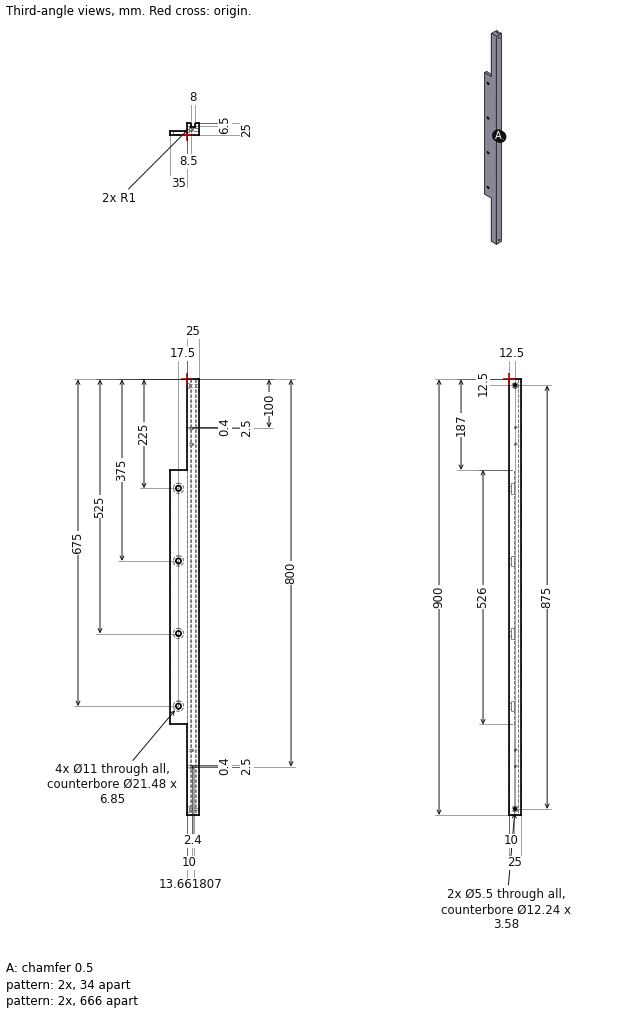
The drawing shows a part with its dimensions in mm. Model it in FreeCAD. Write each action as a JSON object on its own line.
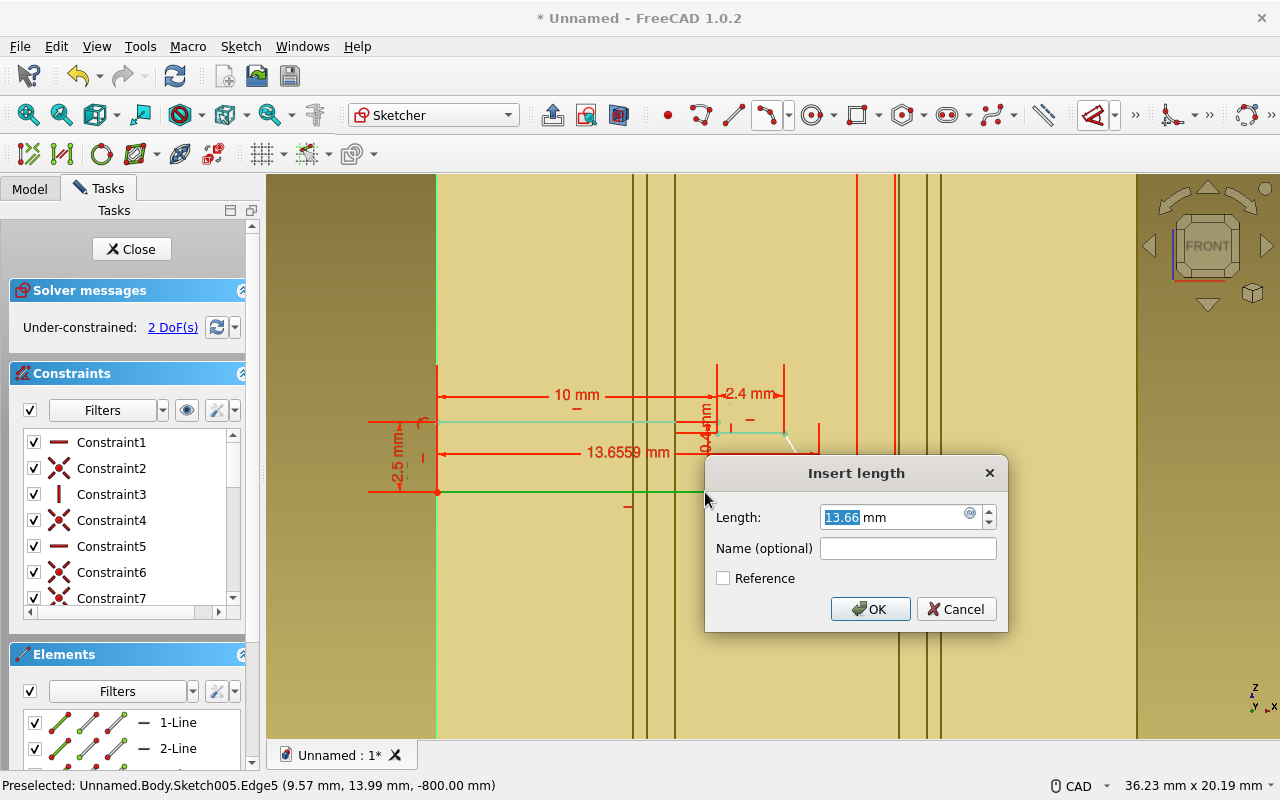
{"action": "type", "text": "13.661807"}
{"action": "key", "text": "Return"}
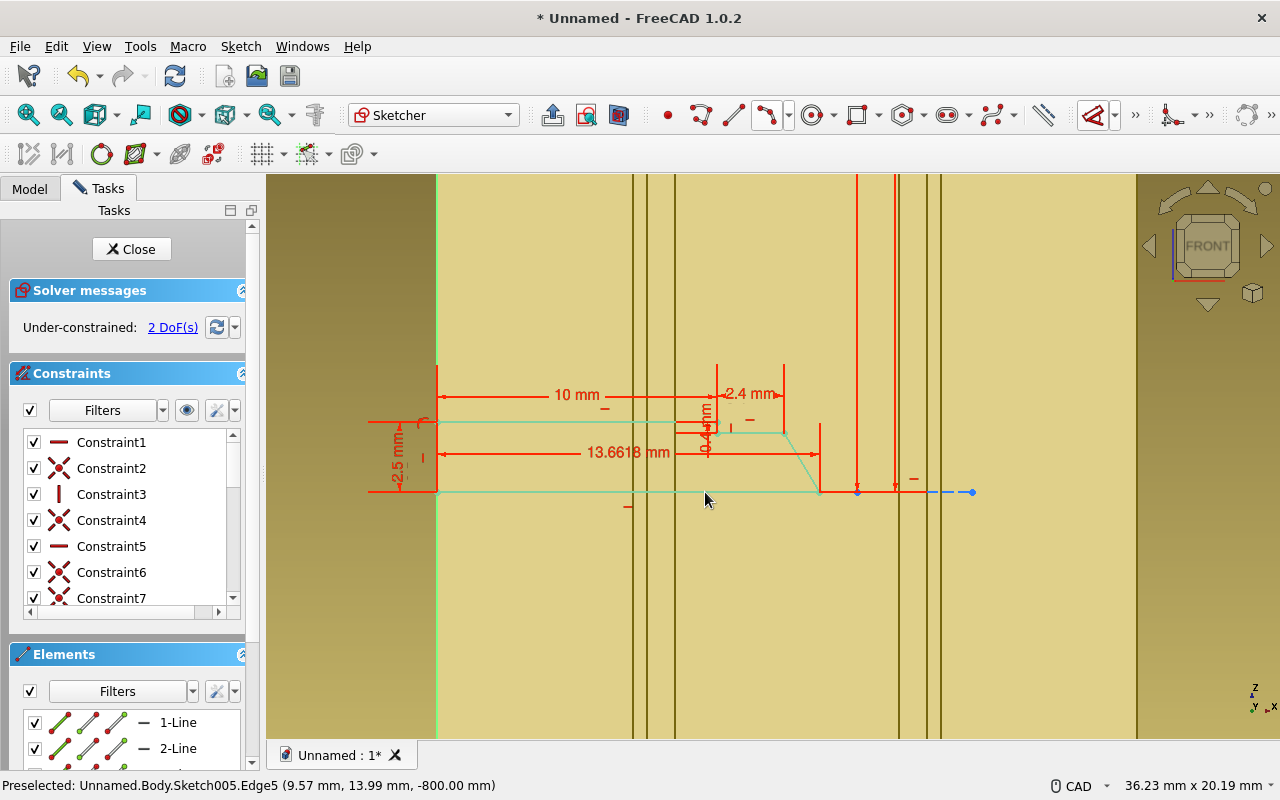
{"action": "left_click", "coordinate": [132, 249]}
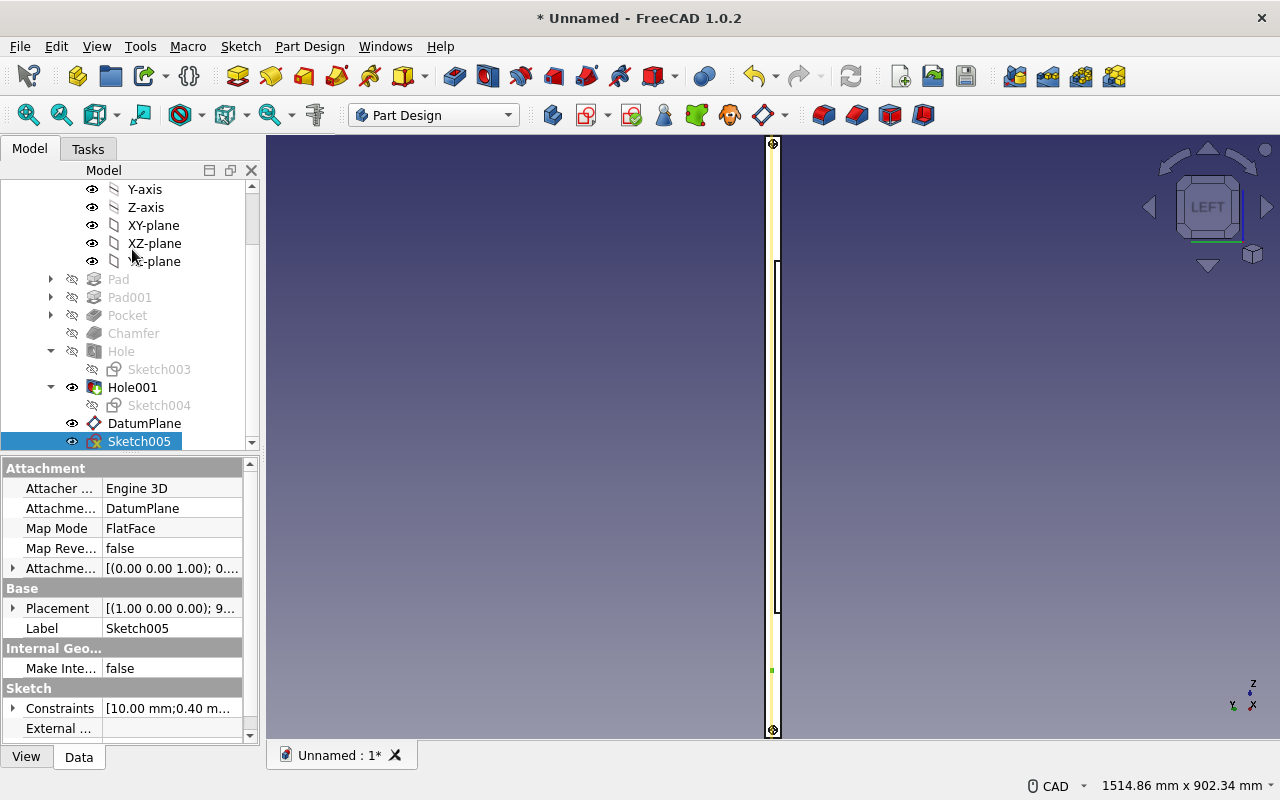
{"action": "left_click", "coordinate": [521, 76]}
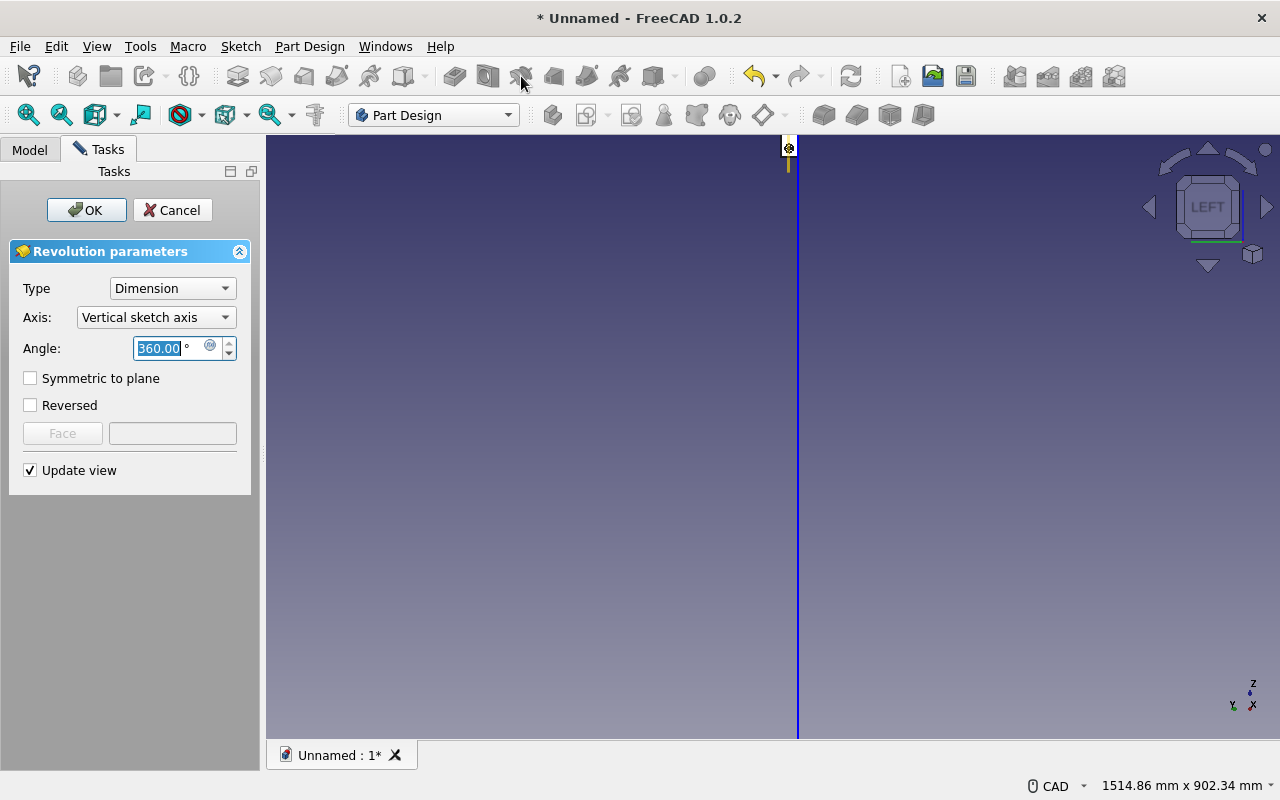
{"action": "left_click", "coordinate": [157, 318]}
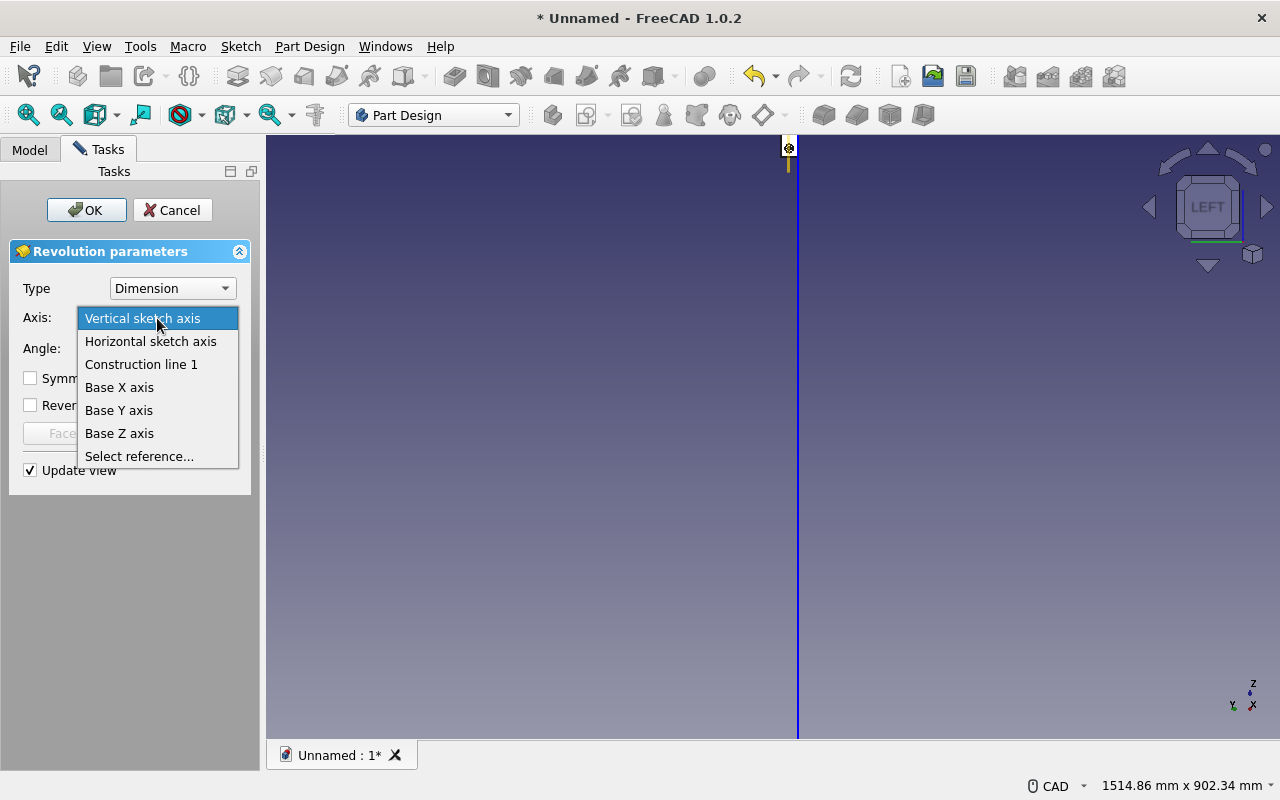
{"action": "left_click", "coordinate": [156, 364]}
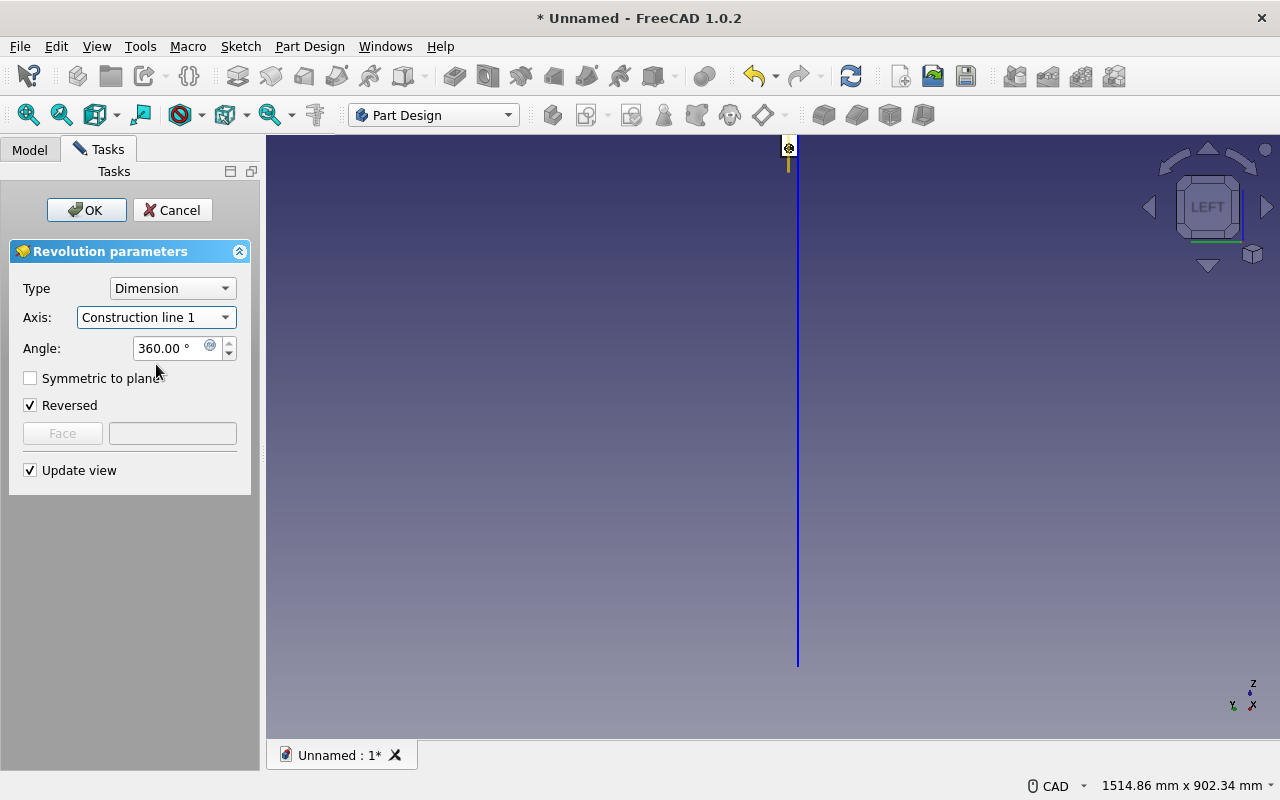
{"action": "left_click", "coordinate": [87, 210]}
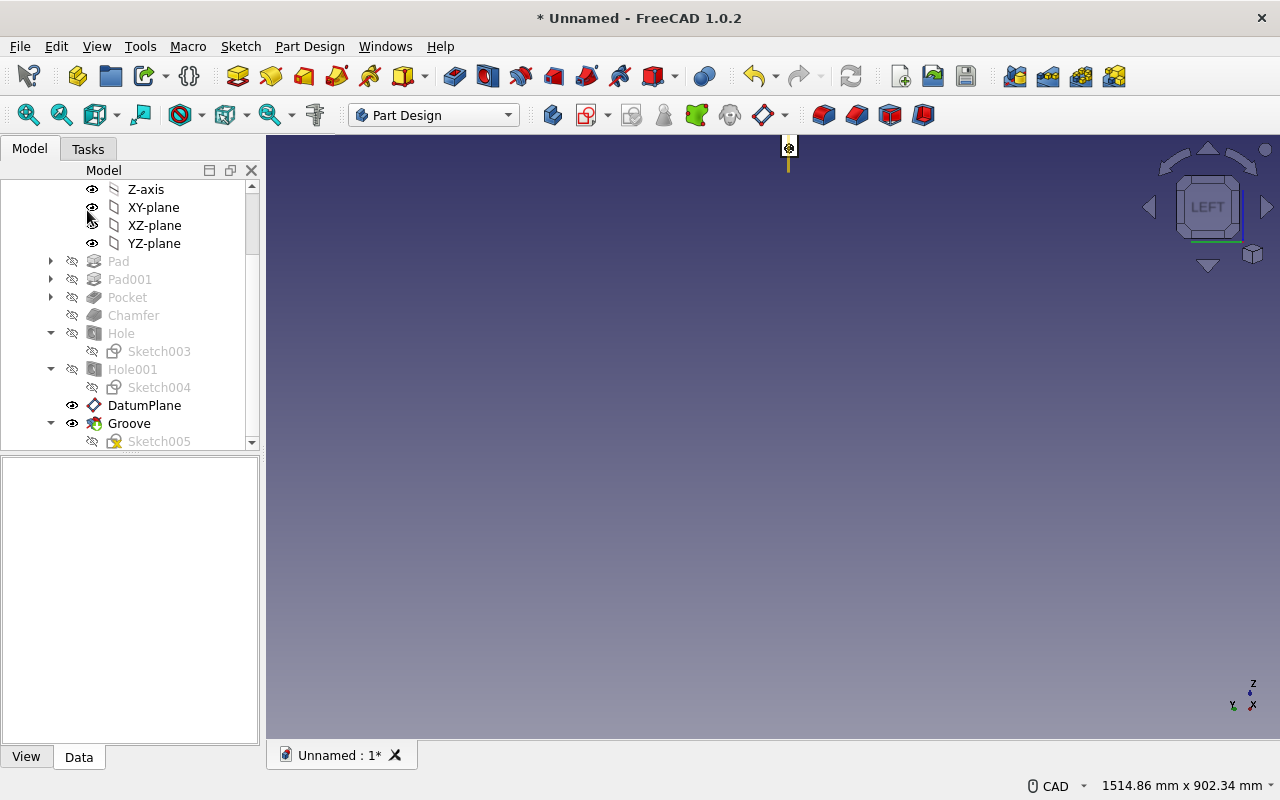
{"action": "left_click", "coordinate": [117, 405]}
{"action": "key", "text": "space"}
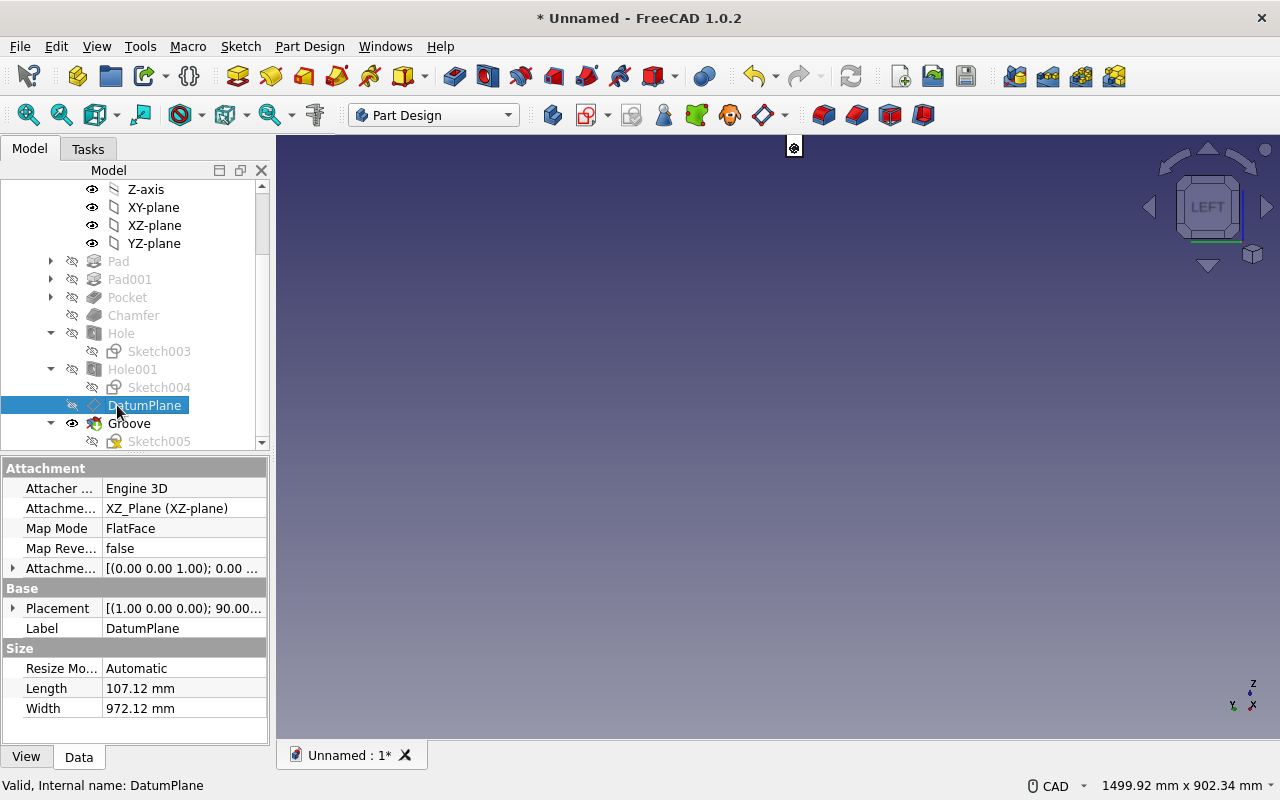
{"action": "left_click", "coordinate": [29, 116]}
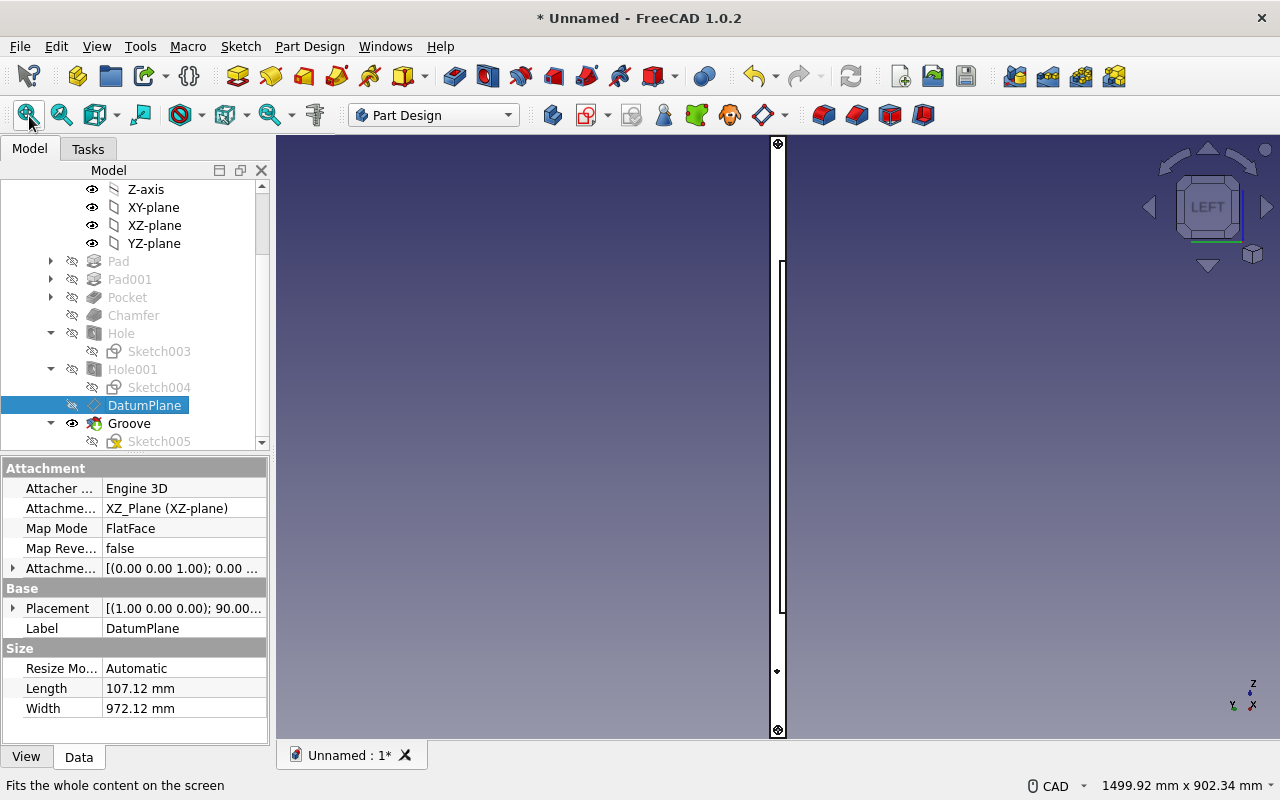
{"action": "left_click", "coordinate": [117, 423]}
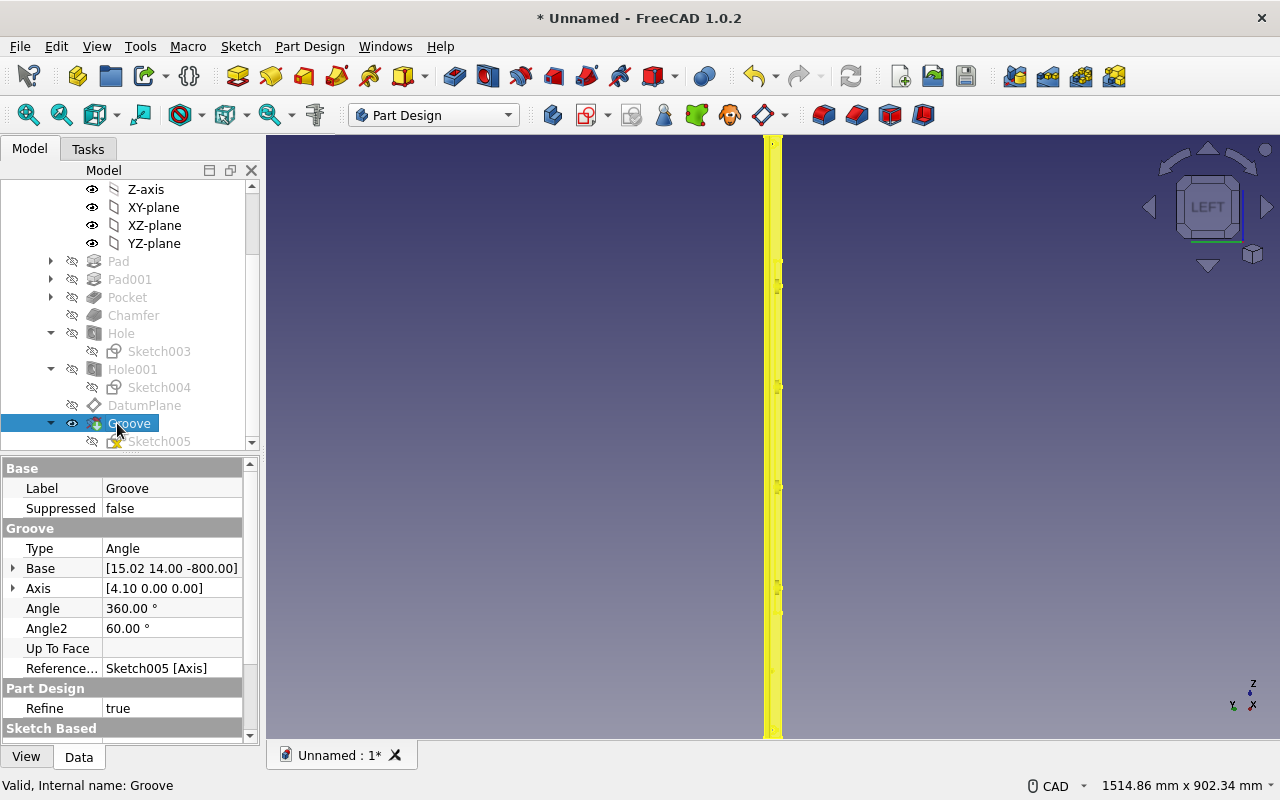
{"action": "left_click", "coordinate": [1048, 76]}